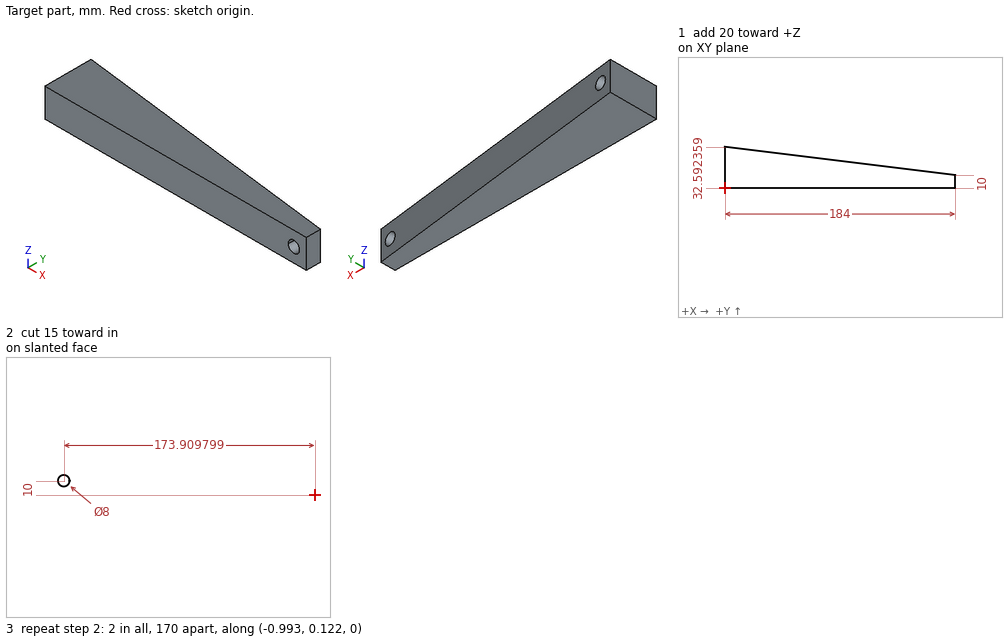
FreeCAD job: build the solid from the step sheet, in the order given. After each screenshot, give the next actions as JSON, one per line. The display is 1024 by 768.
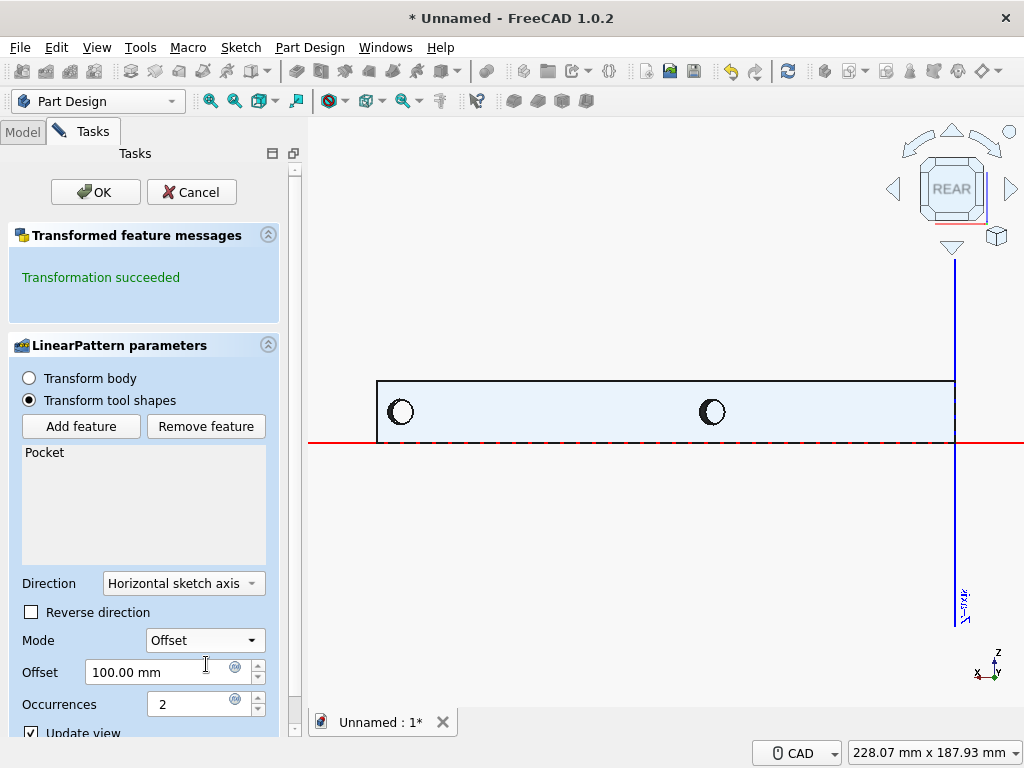
{"action": "triple_click", "coordinate": [168, 672]}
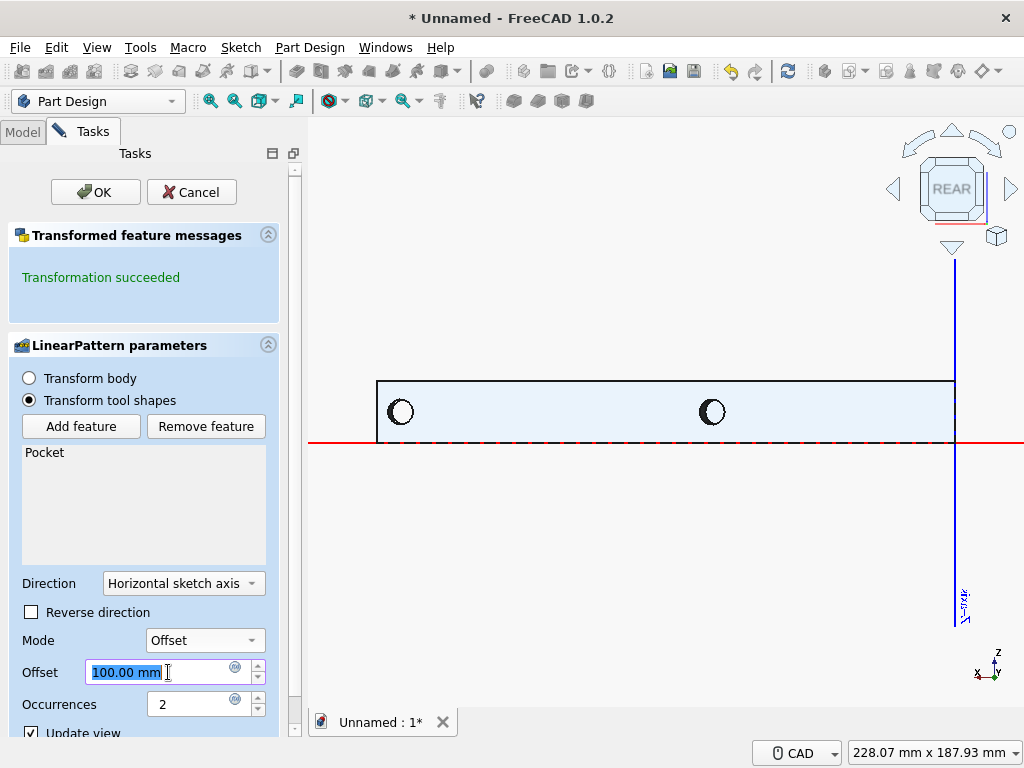
{"action": "type", "text": "170"}
{"action": "key", "text": "Tab"}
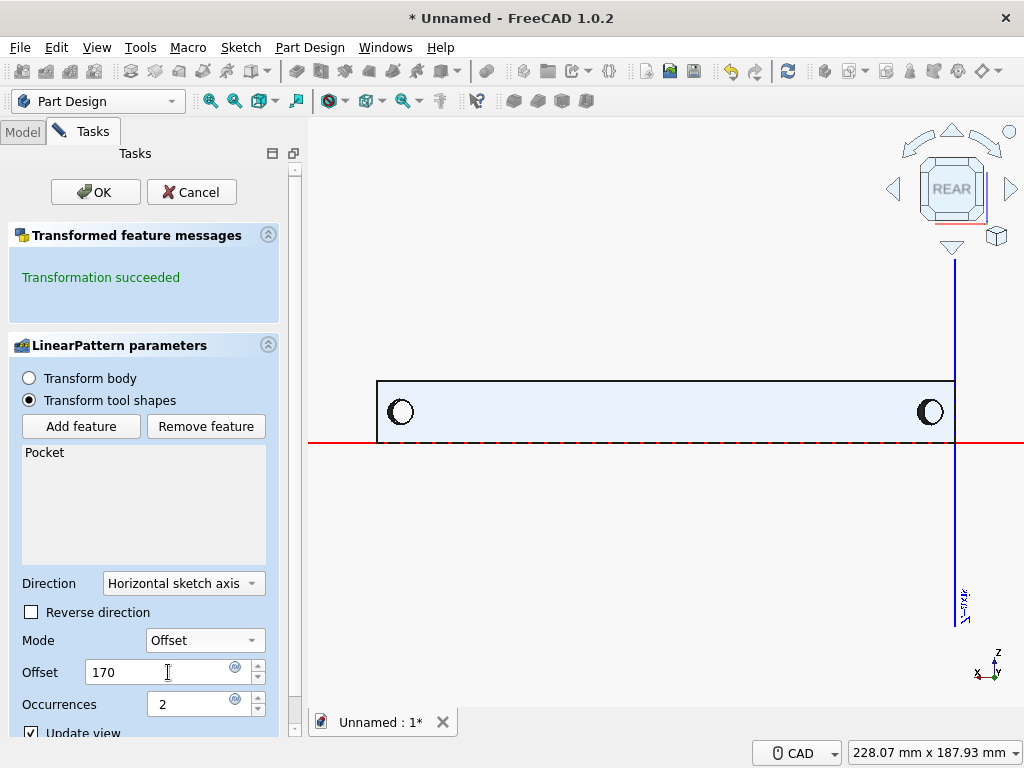
{"action": "triple_click", "coordinate": [198, 704]}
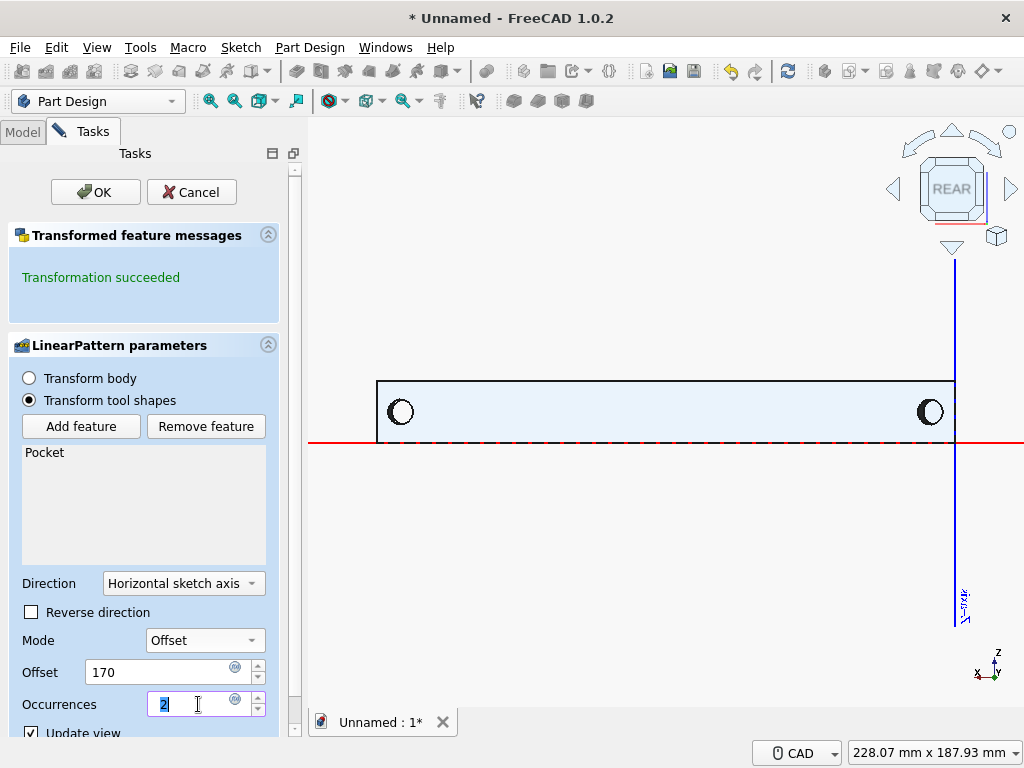
{"action": "type", "text": "2"}
{"action": "key", "text": "Tab"}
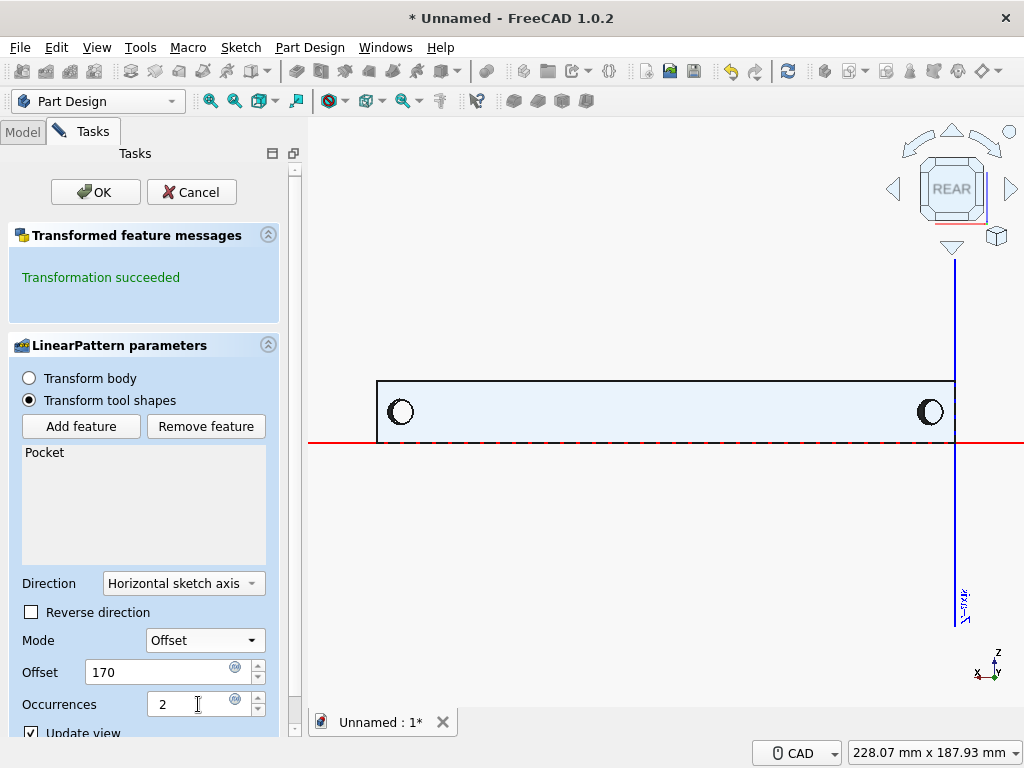
{"action": "left_click", "coordinate": [96, 192]}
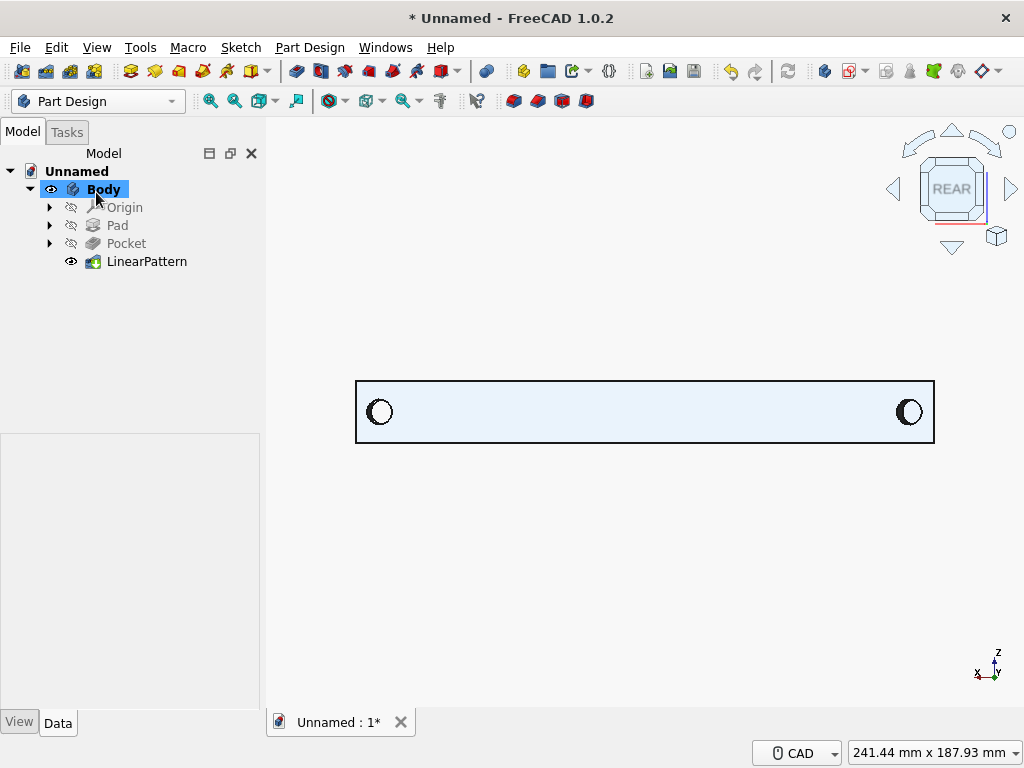
{"action": "key", "text": "0"}